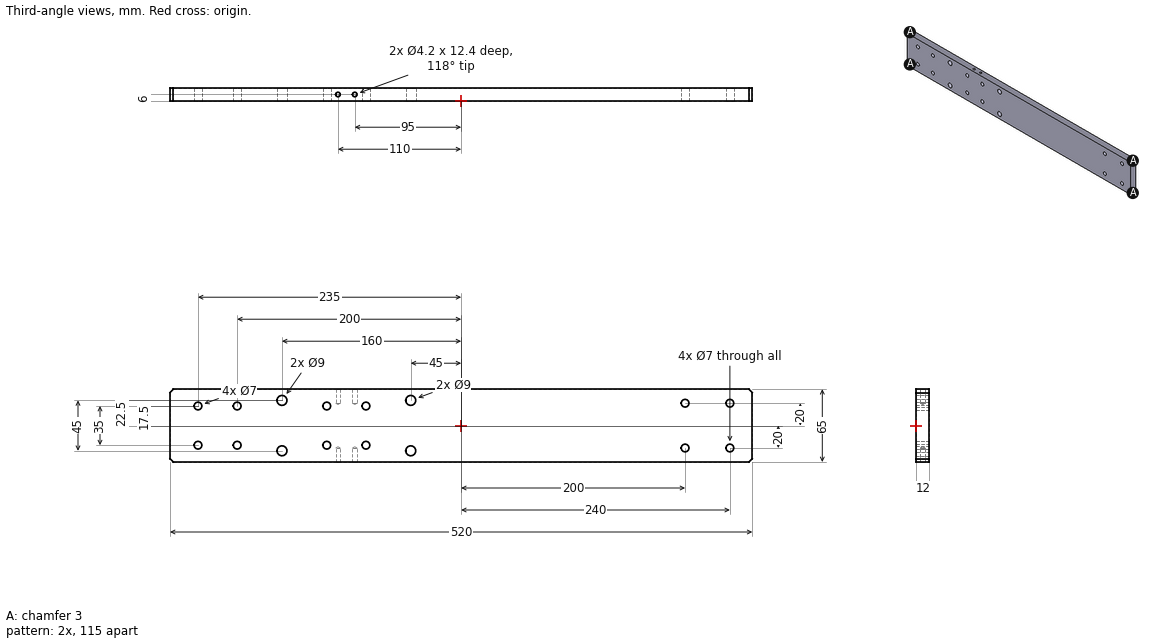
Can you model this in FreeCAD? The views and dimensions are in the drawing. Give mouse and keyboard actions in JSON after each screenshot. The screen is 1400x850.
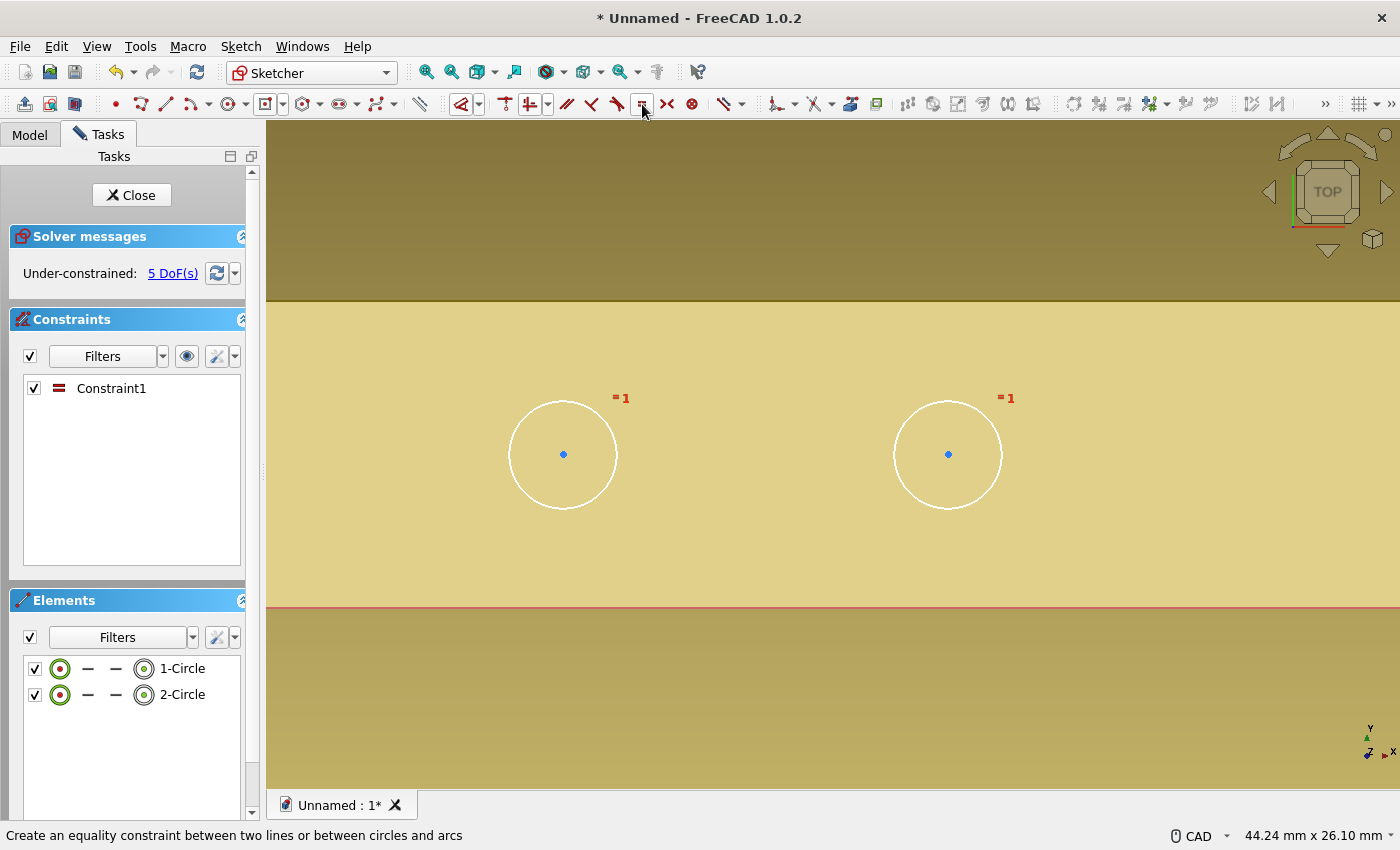
{"action": "left_click", "coordinate": [948, 455]}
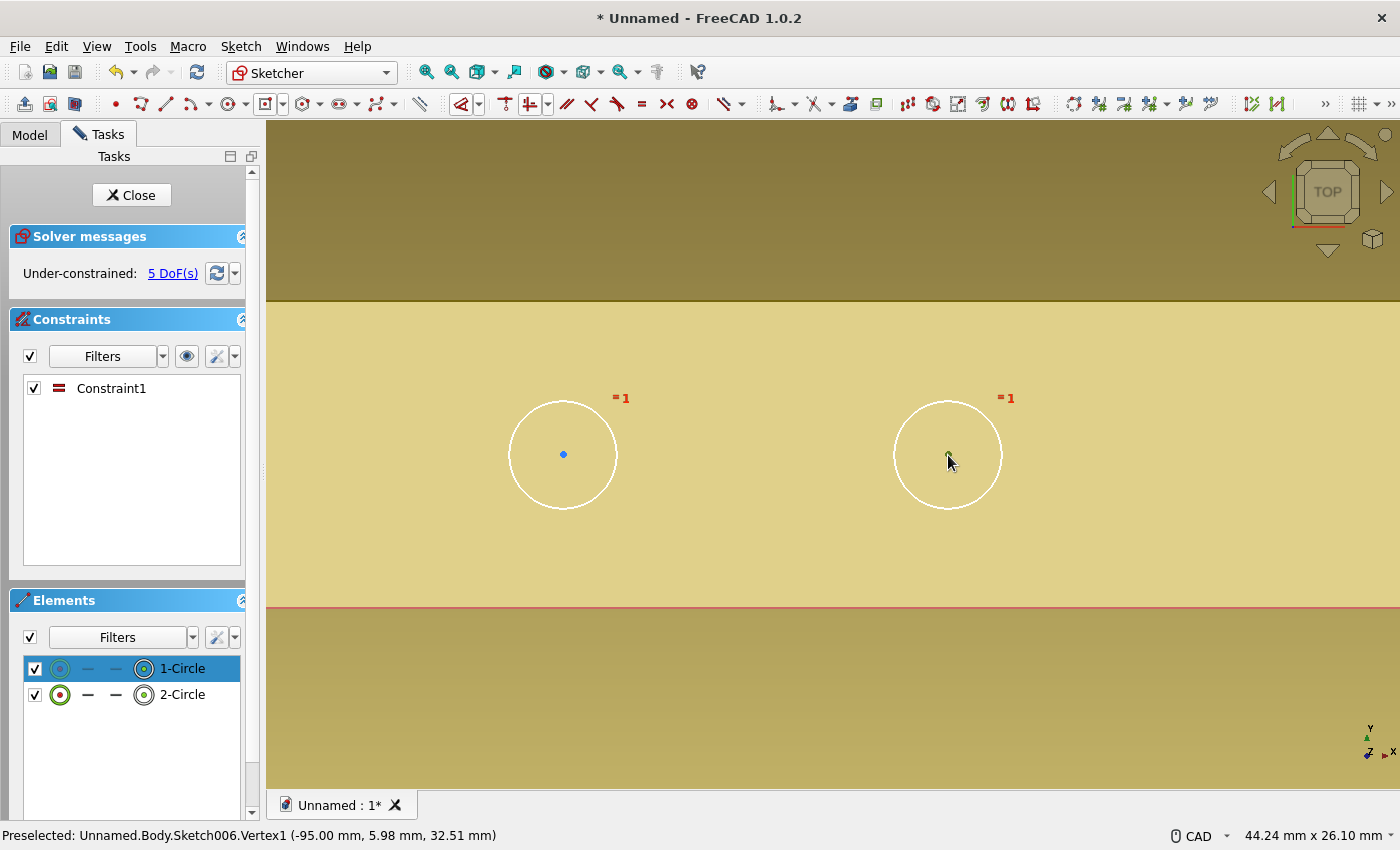
{"action": "left_click", "coordinate": [563, 455]}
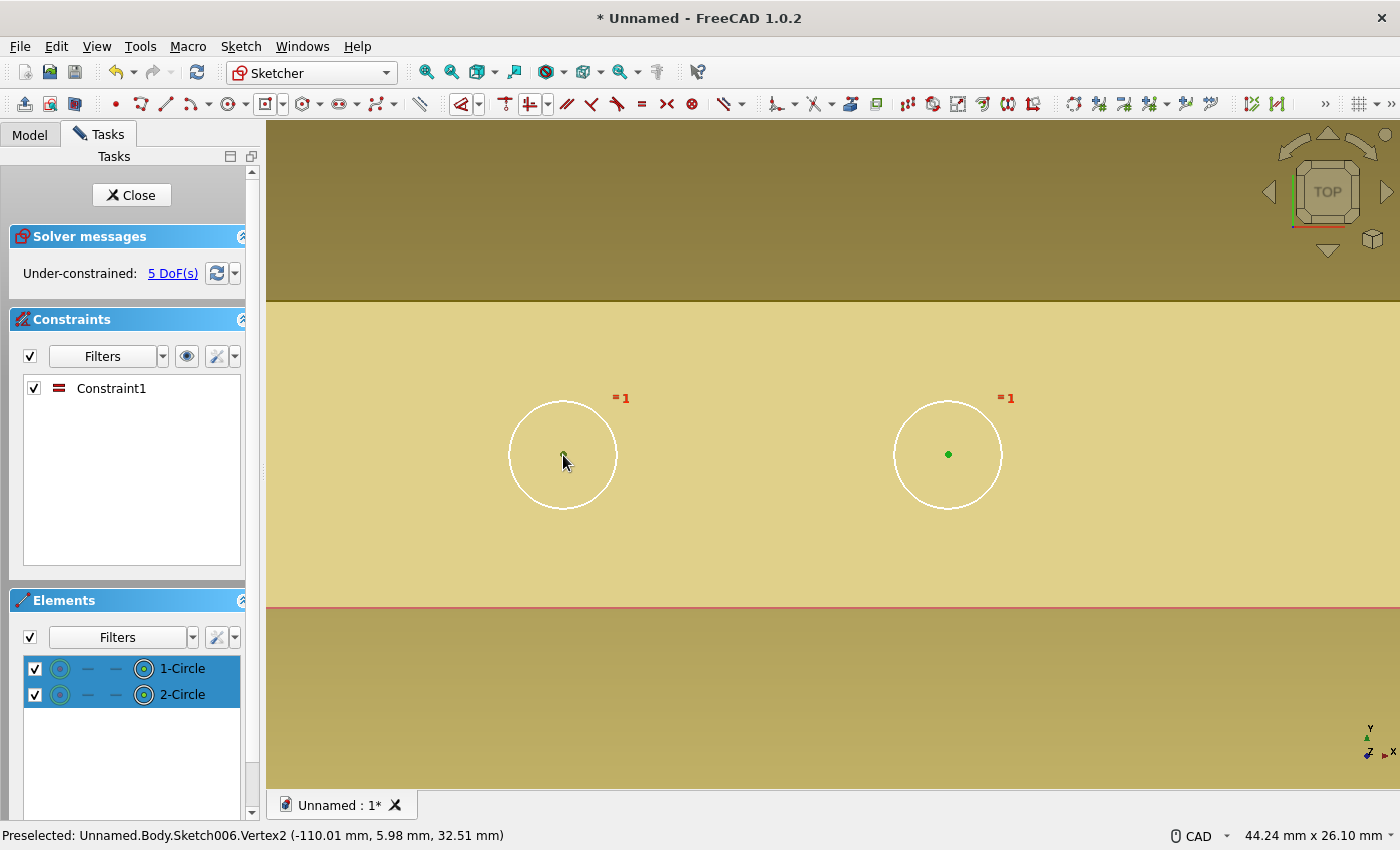
{"action": "left_click", "coordinate": [548, 104]}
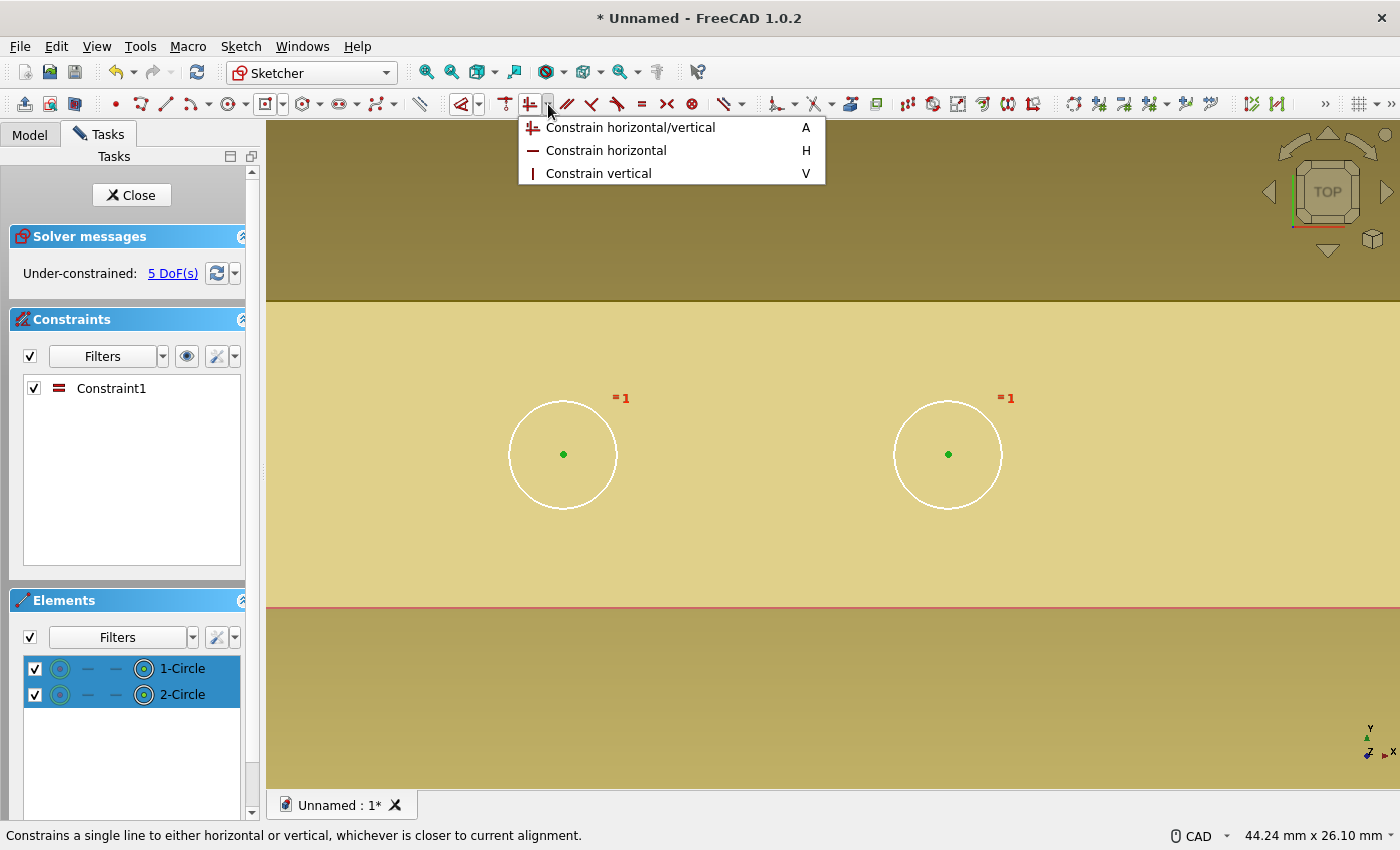
{"action": "left_click", "coordinate": [672, 150]}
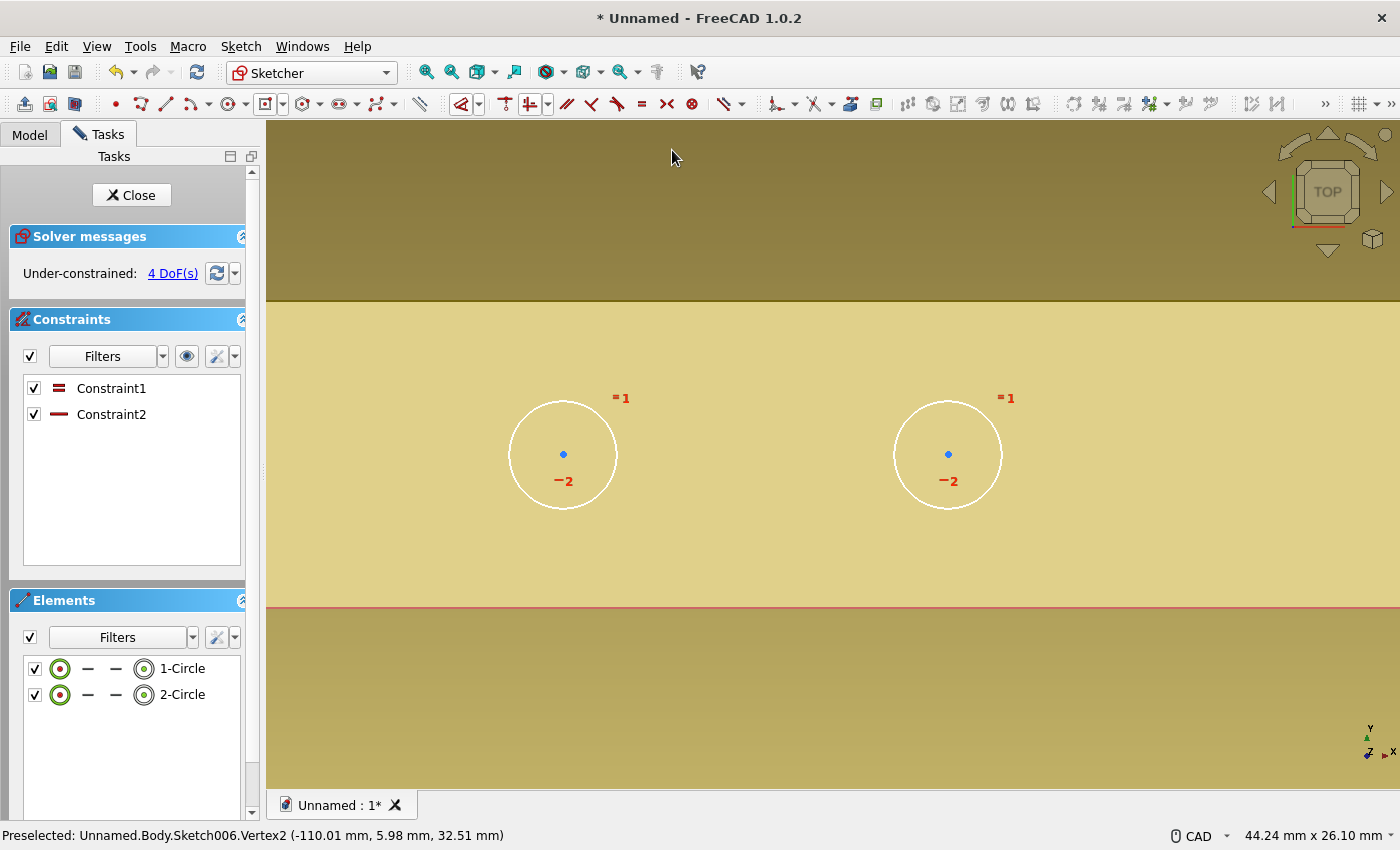
{"action": "left_click", "coordinate": [986, 417]}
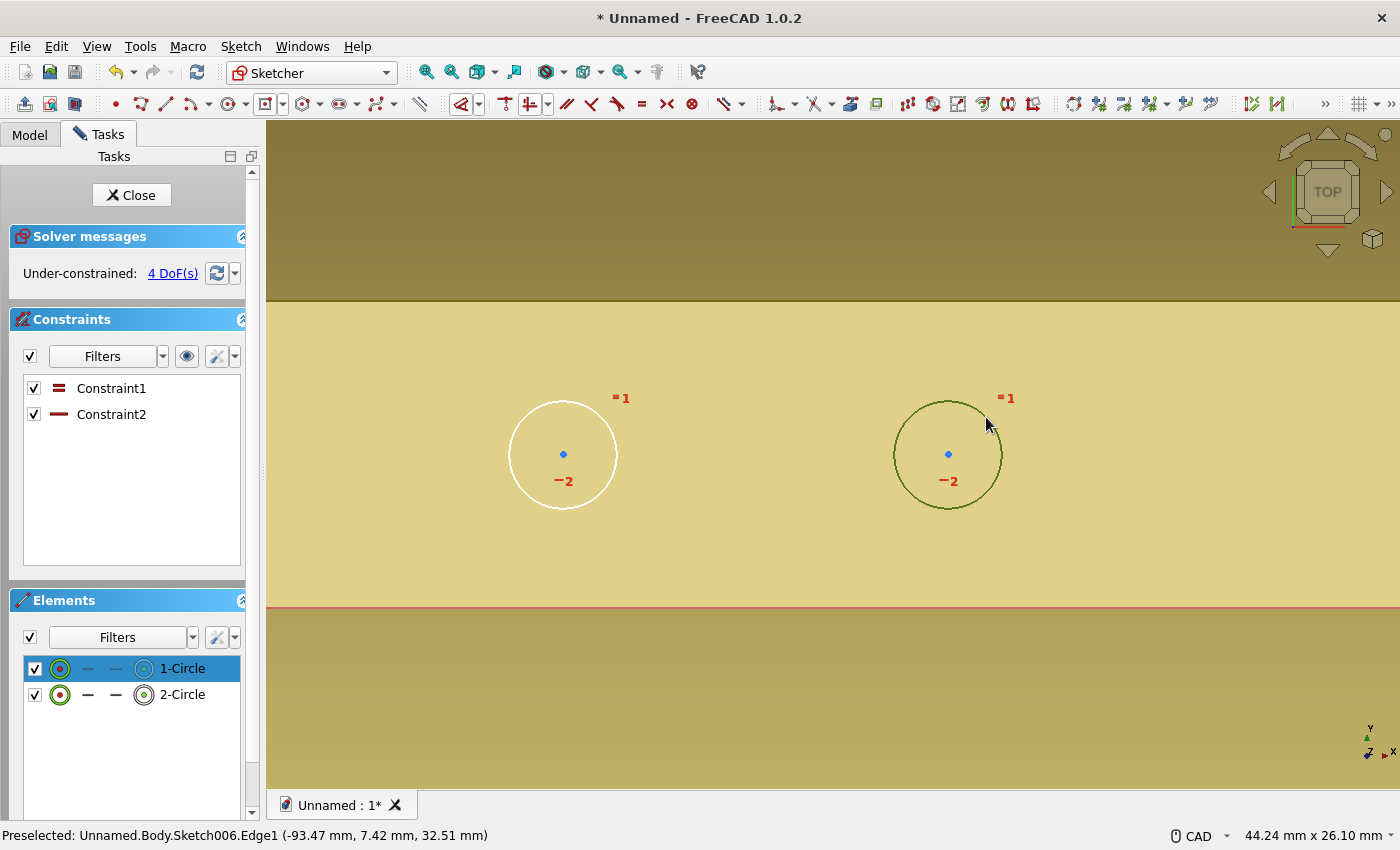
{"action": "left_click", "coordinate": [478, 104]}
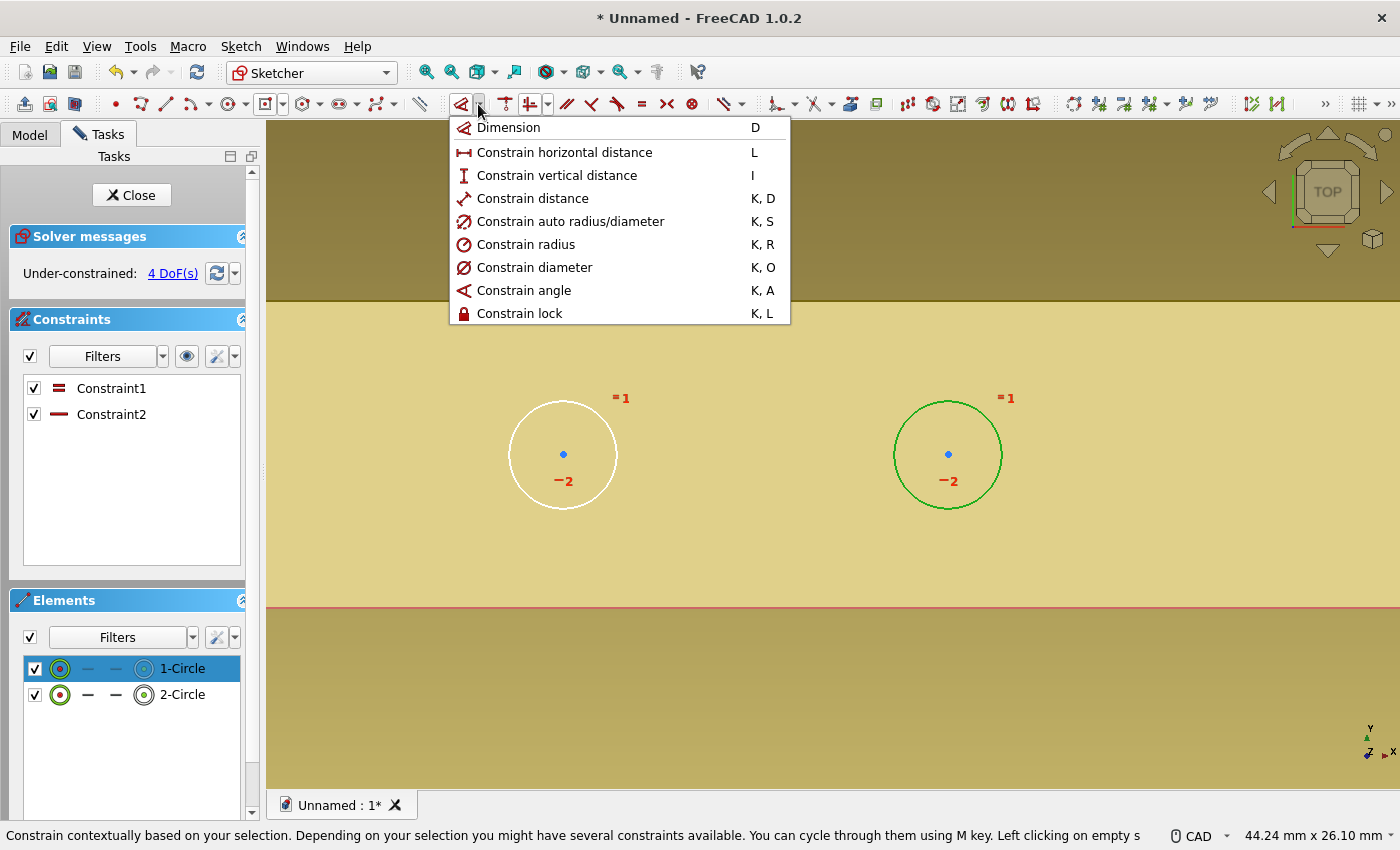
{"action": "left_click", "coordinate": [620, 268]}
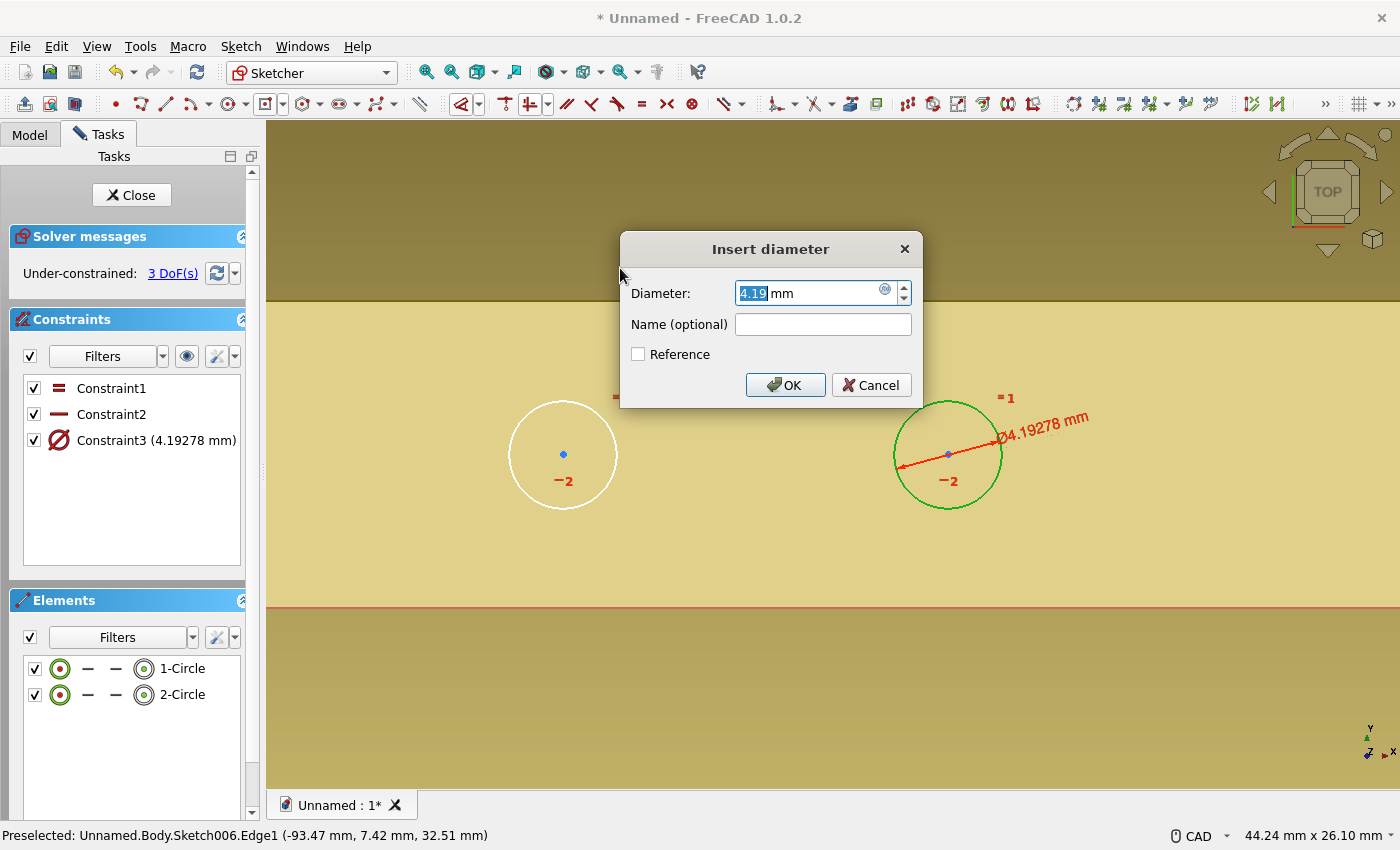
{"action": "type", "text": "4.2"}
{"action": "key", "text": "Return"}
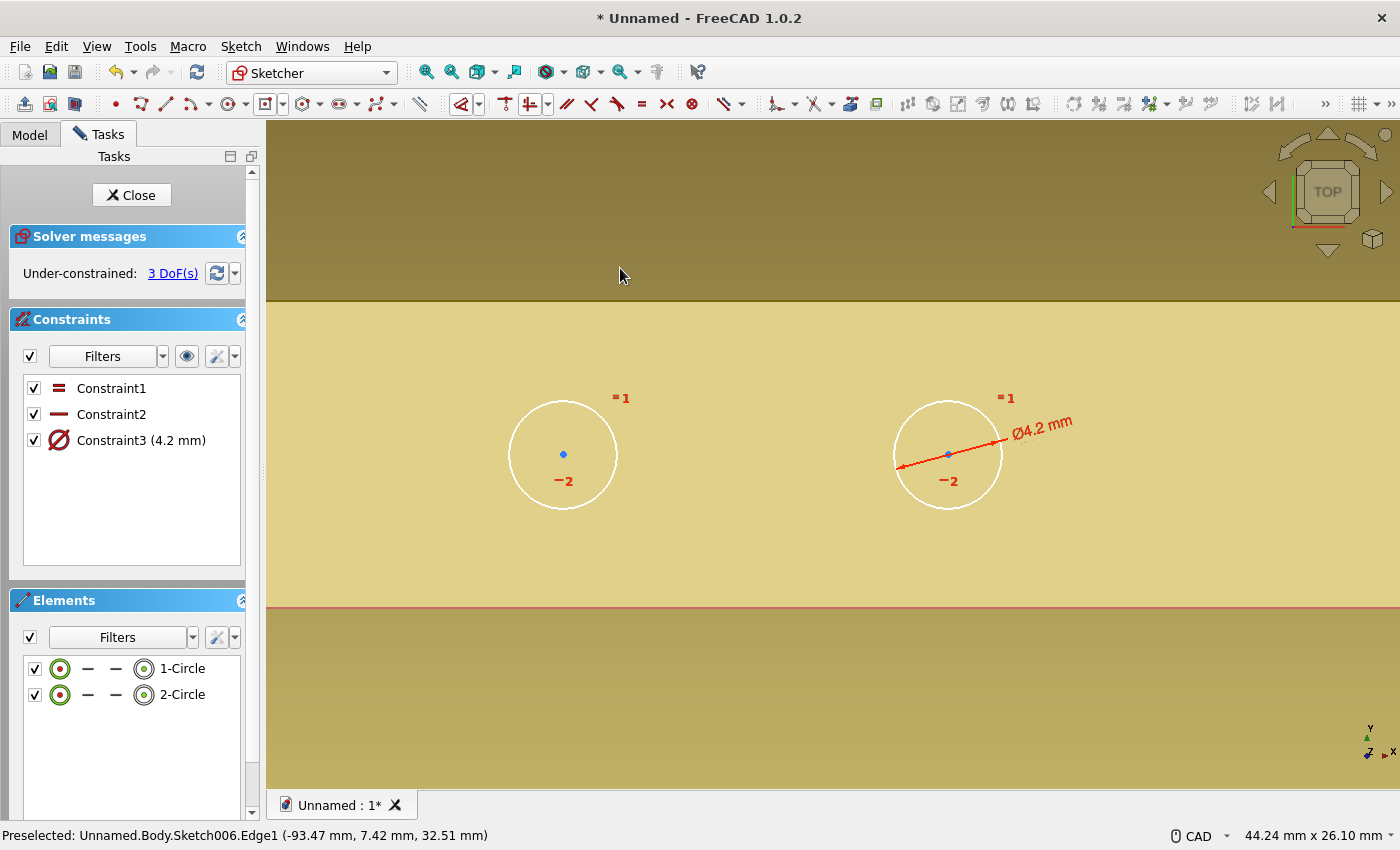
{"action": "left_click", "coordinate": [948, 455]}